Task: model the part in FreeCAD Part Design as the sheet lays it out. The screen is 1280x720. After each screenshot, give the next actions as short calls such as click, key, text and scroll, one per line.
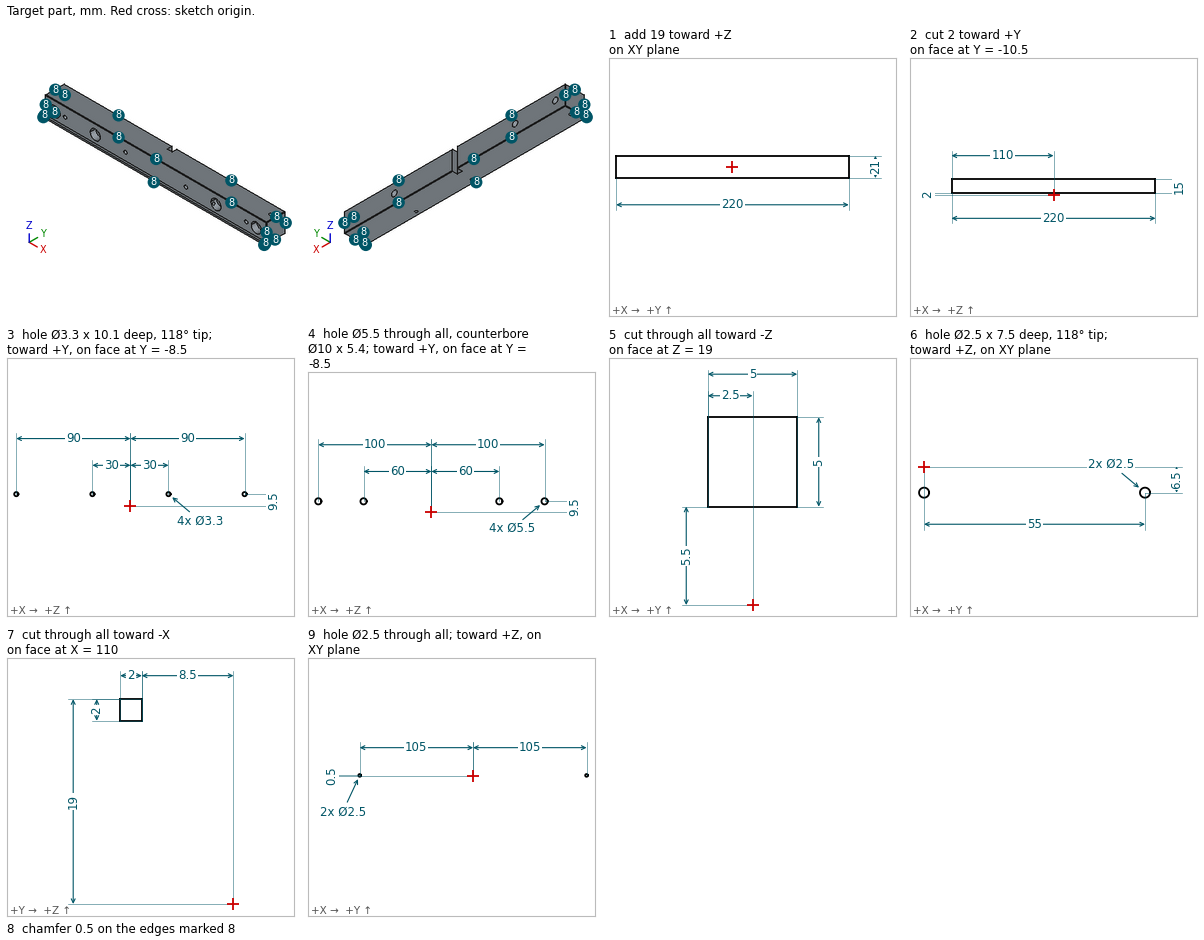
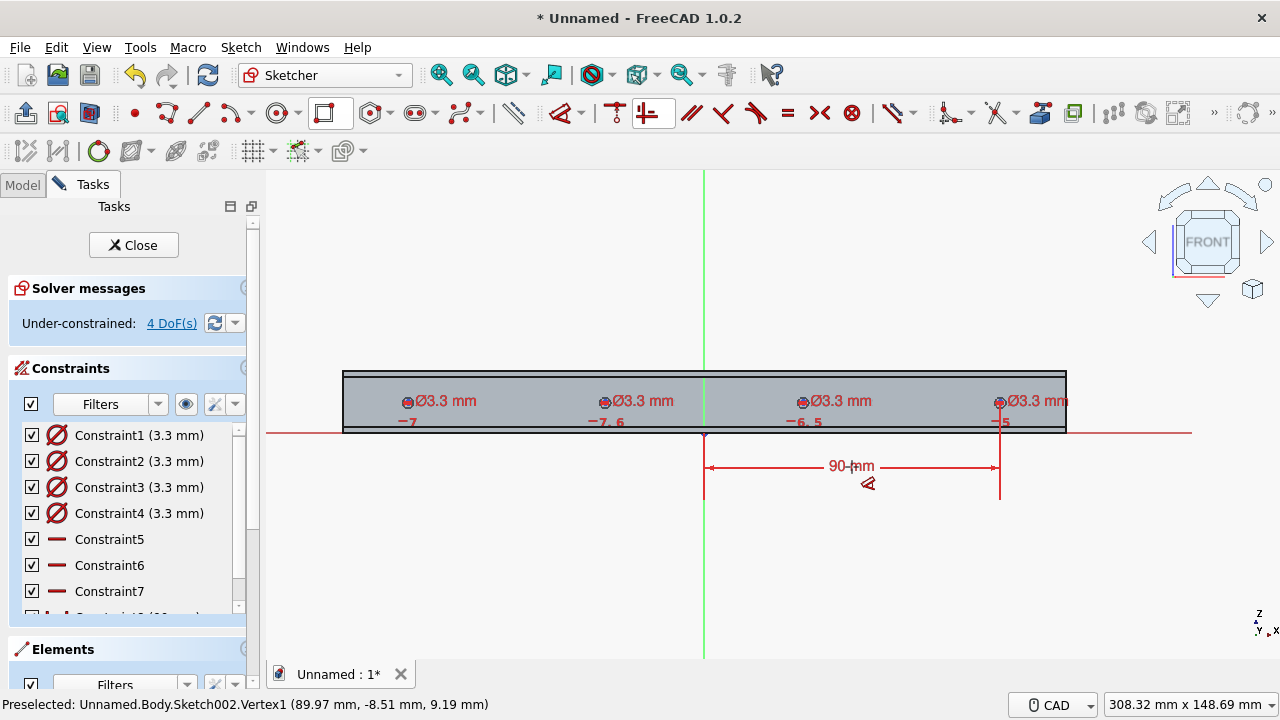
click(803, 403)
click(754, 467)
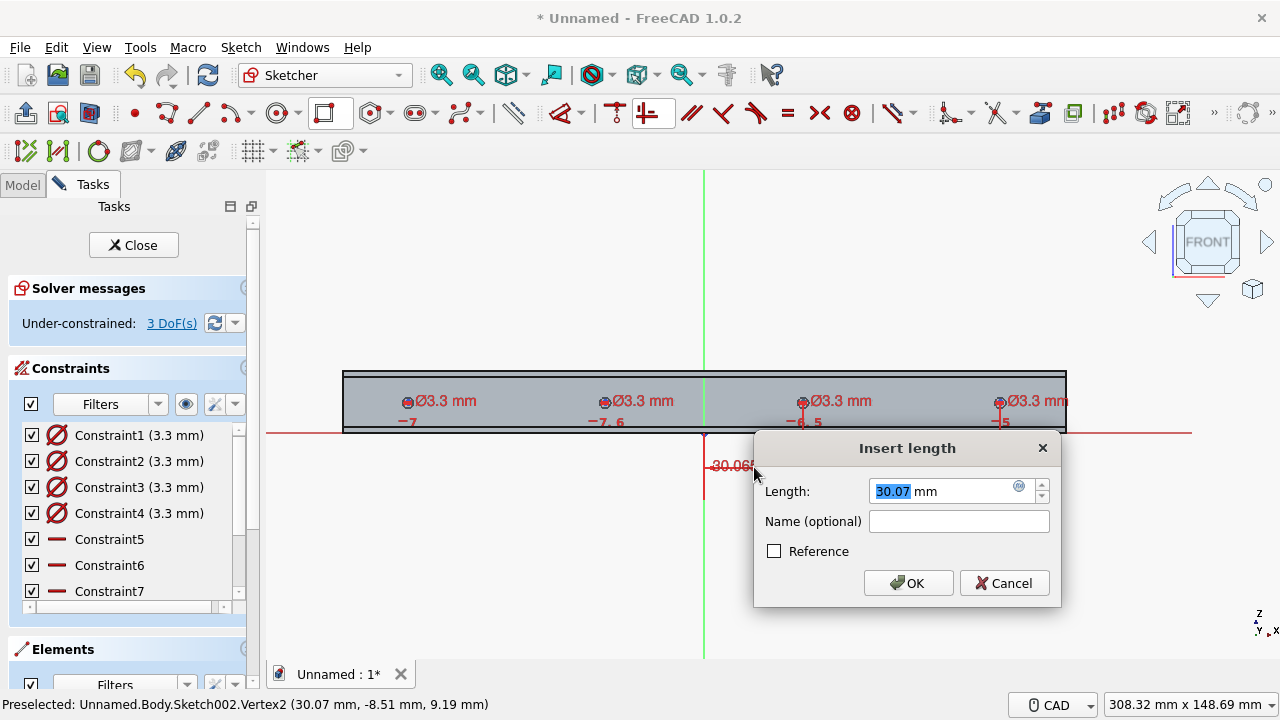
text(30)
key(Return)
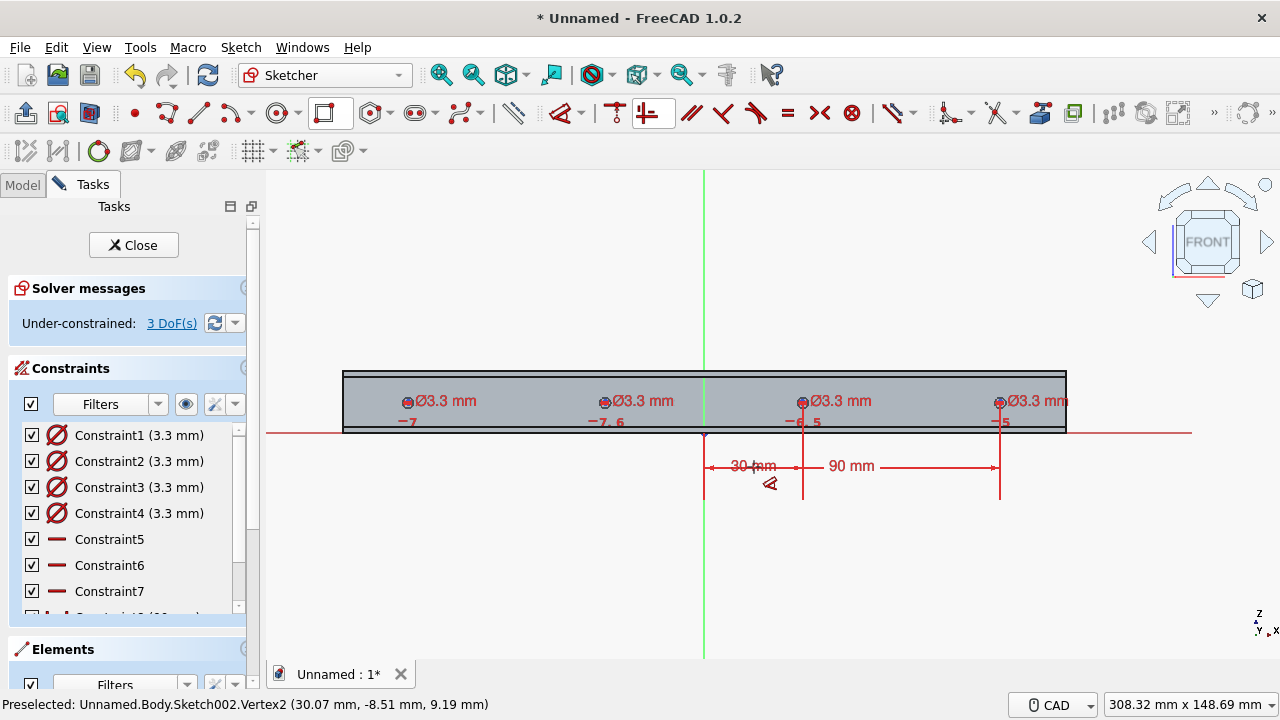
click(605, 403)
click(655, 467)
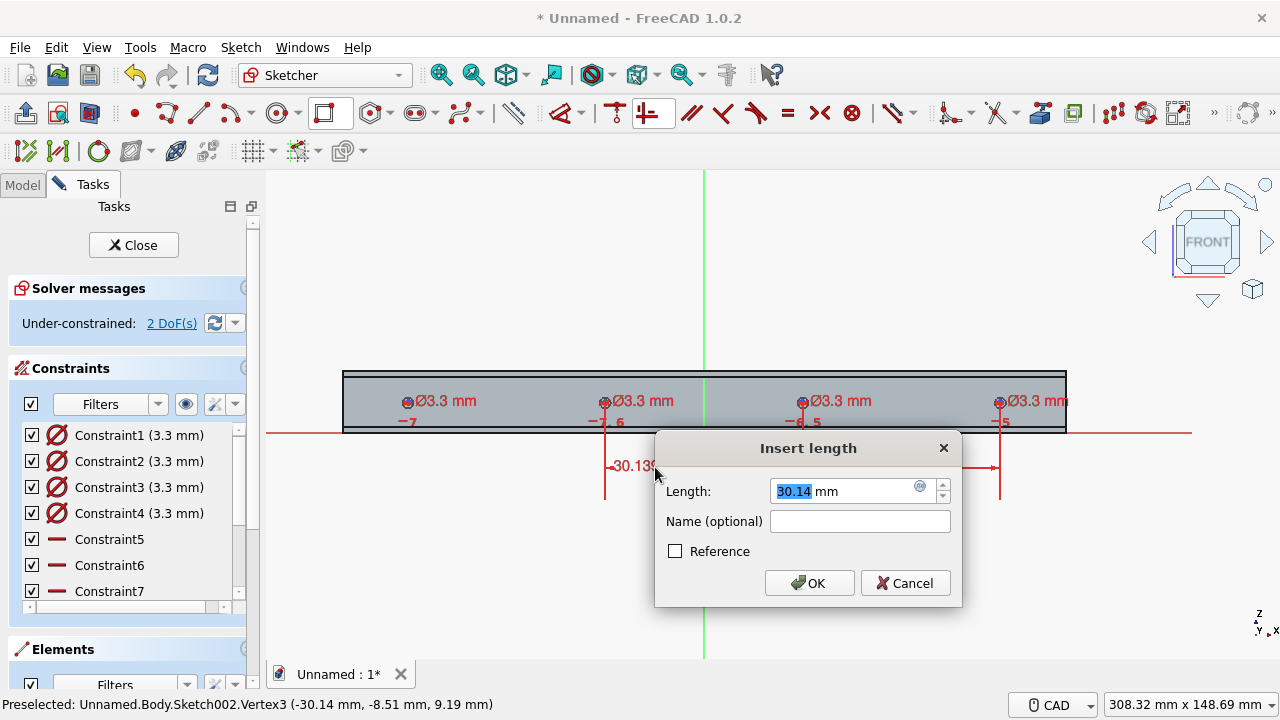
text(30)
key(Return)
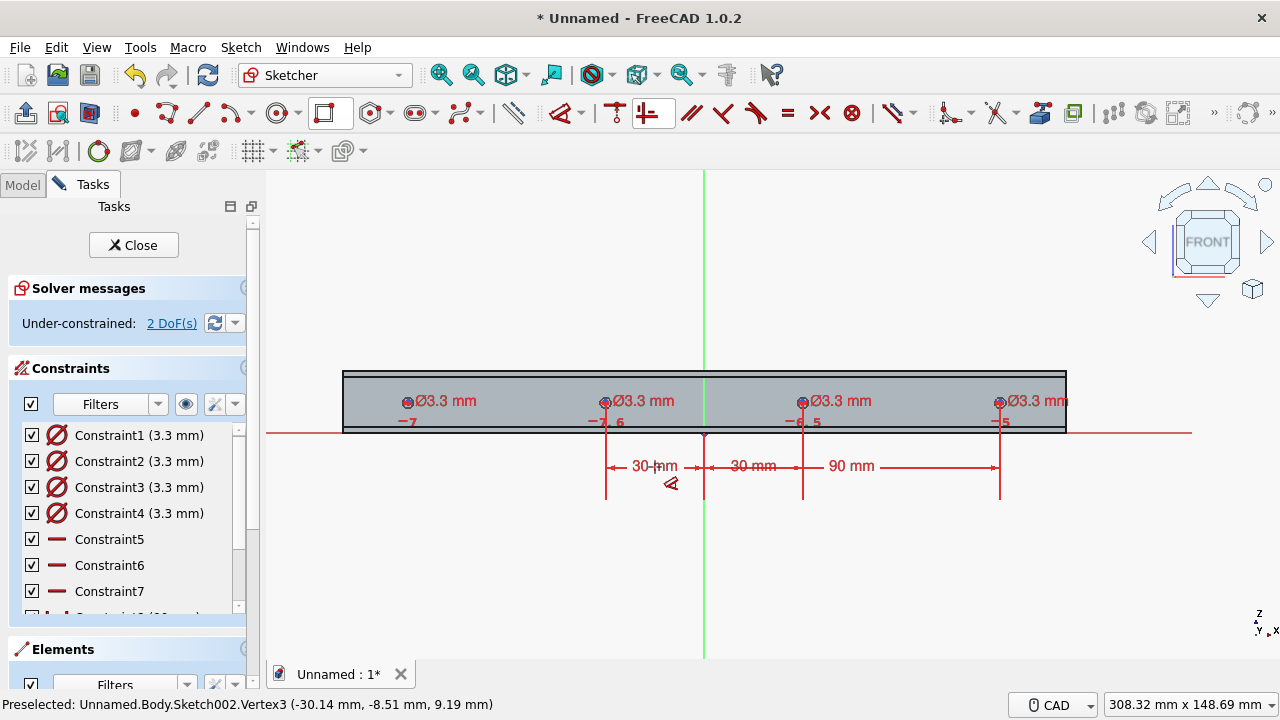
click(408, 403)
click(556, 467)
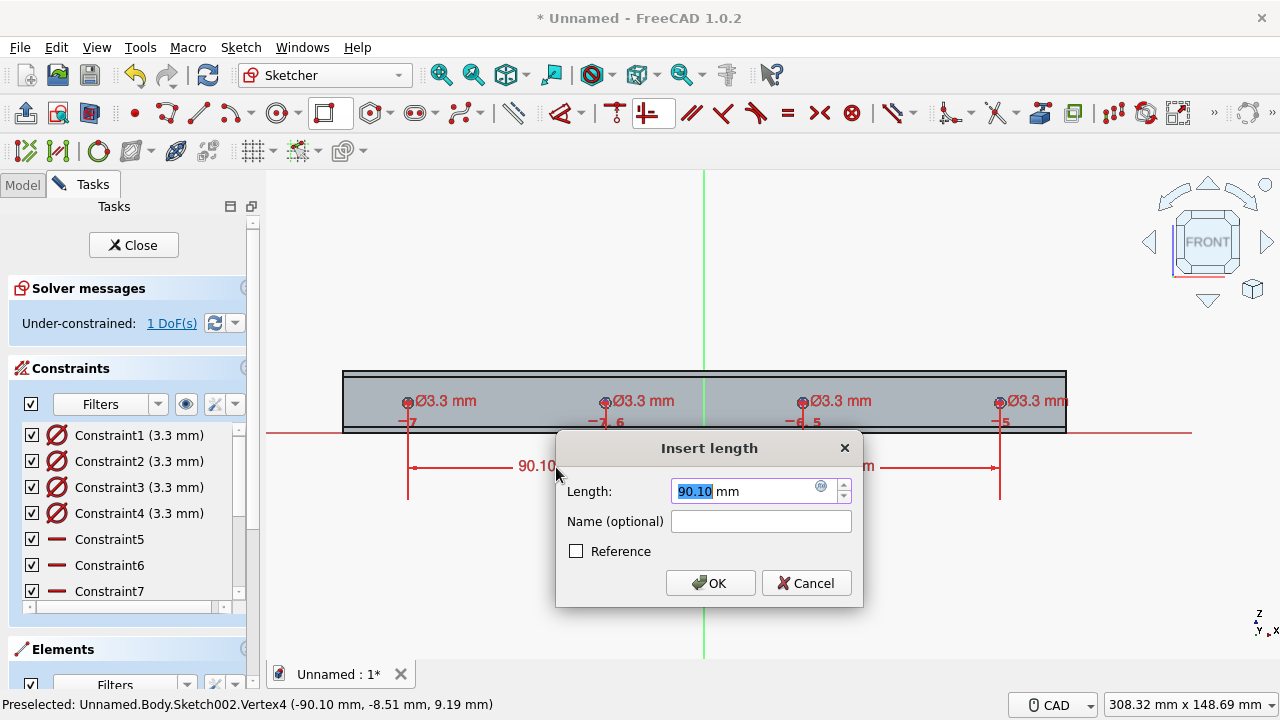
text(90)
key(Return)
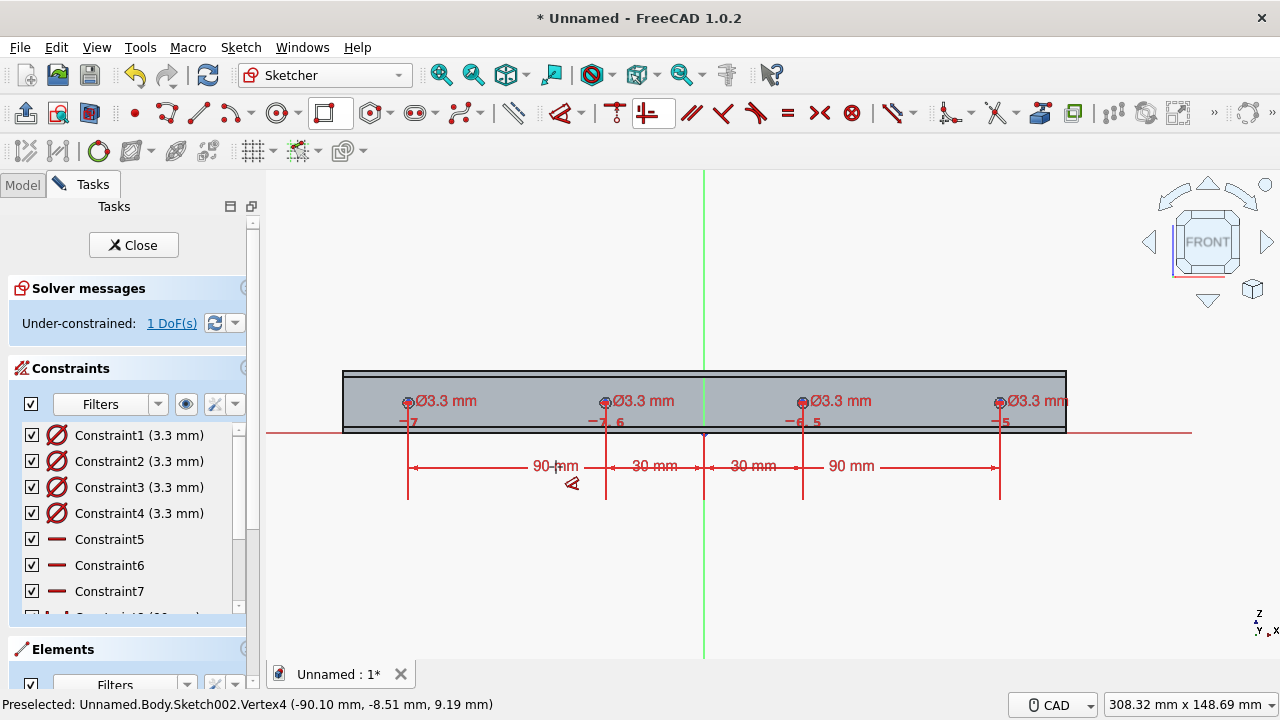
scroll(1000, 403, up, 2)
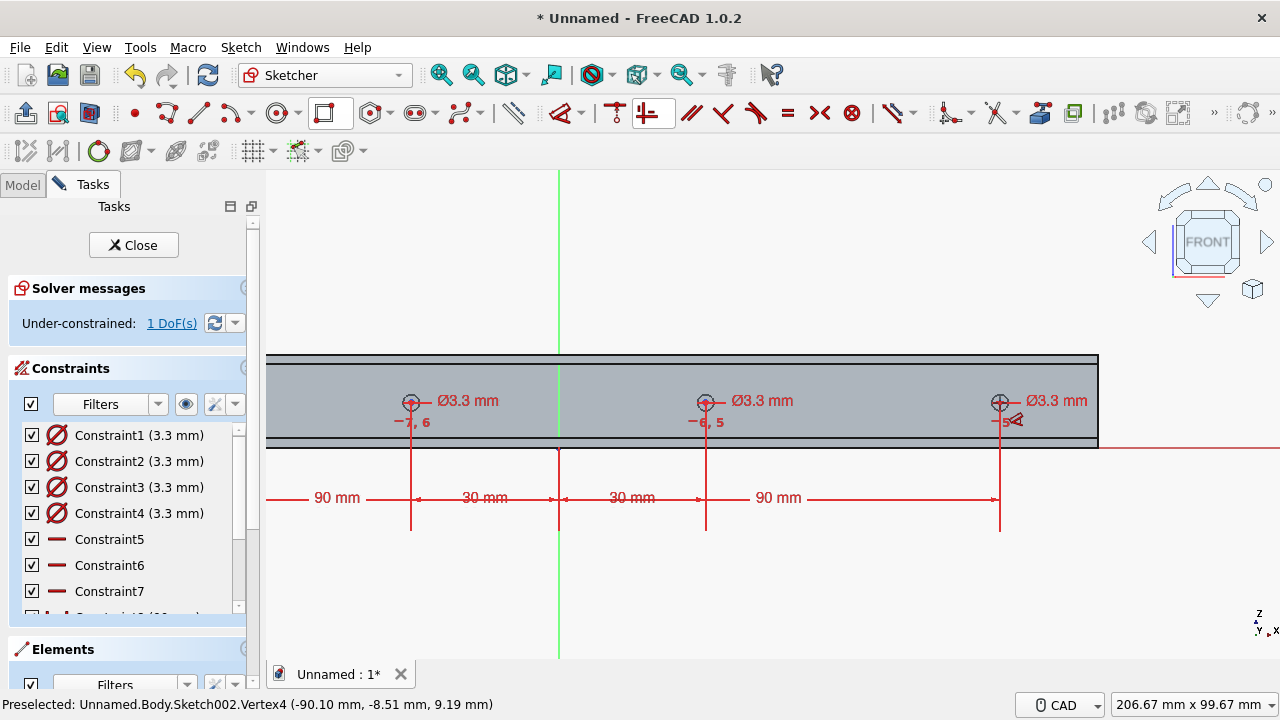
click(1000, 403)
click(1034, 425)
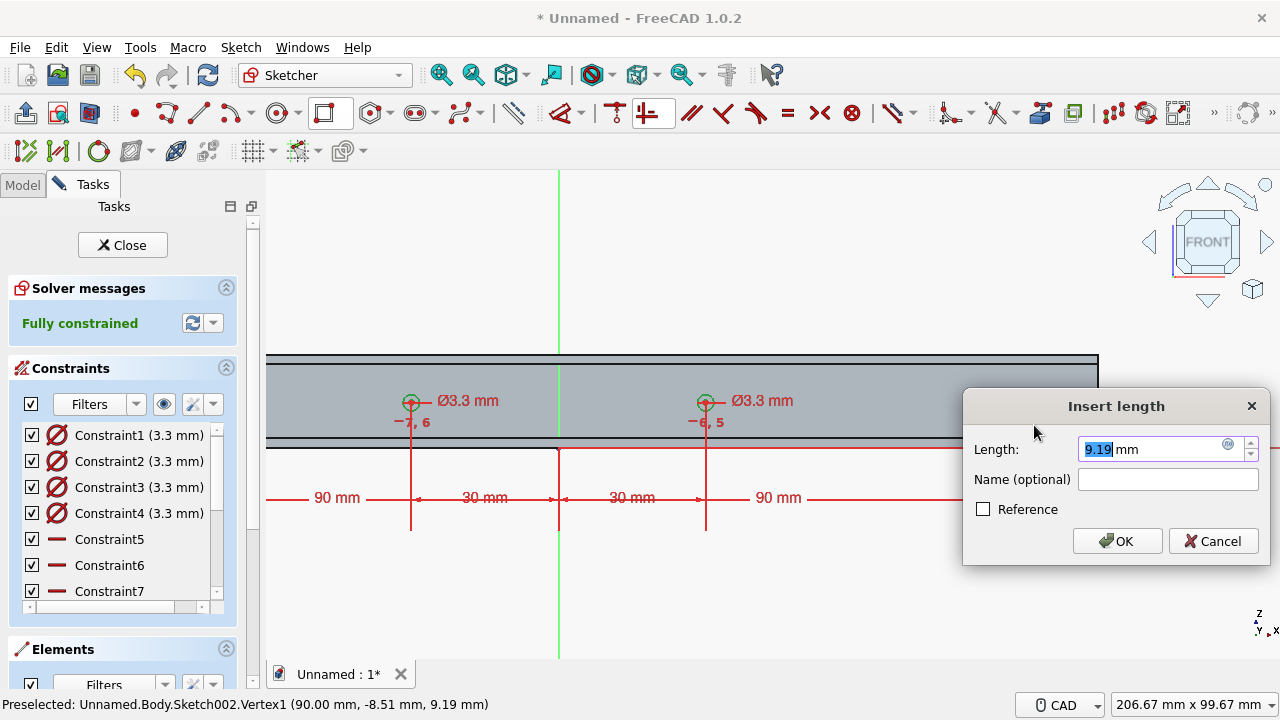
text(9.5)
key(Return)
key(Escape)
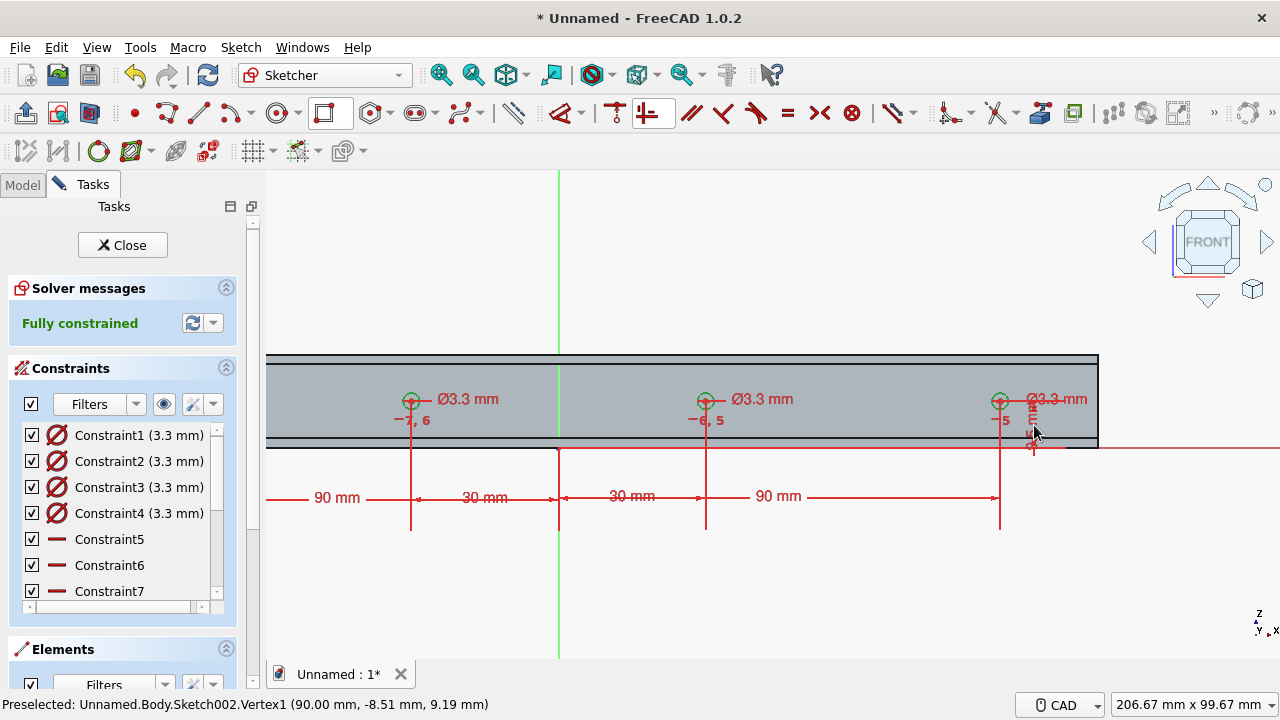
click(123, 245)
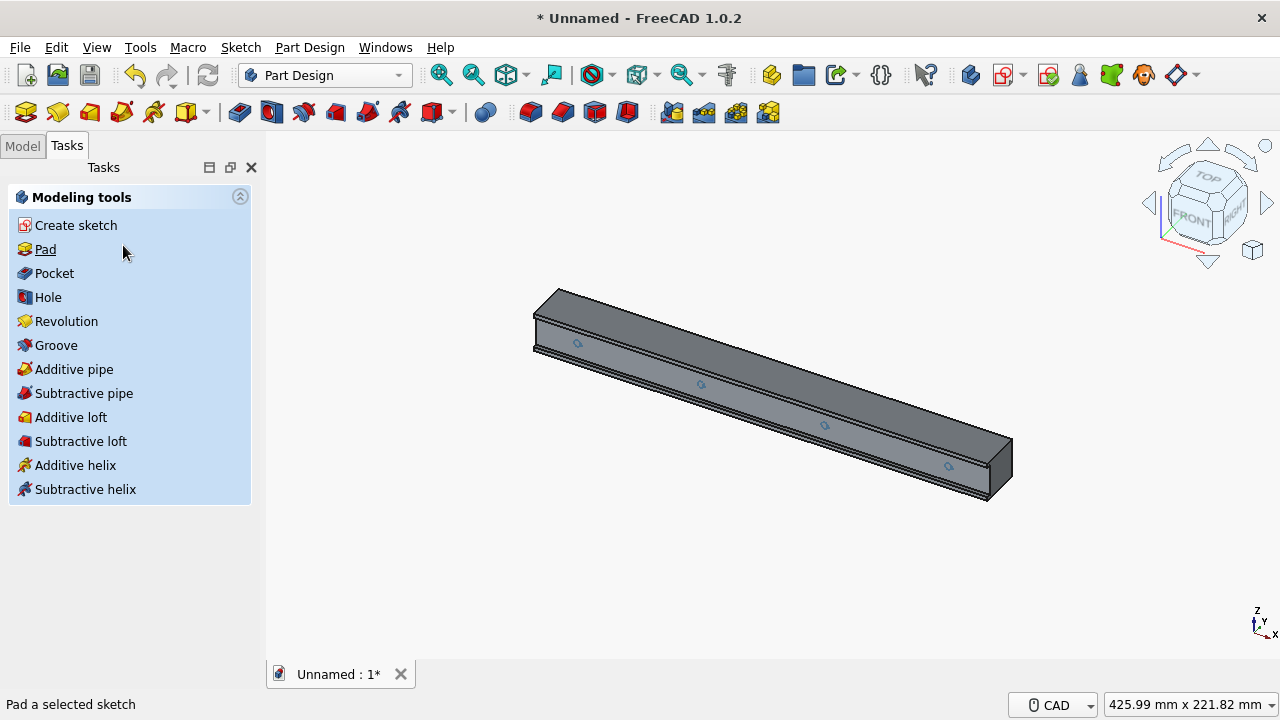
click(272, 112)